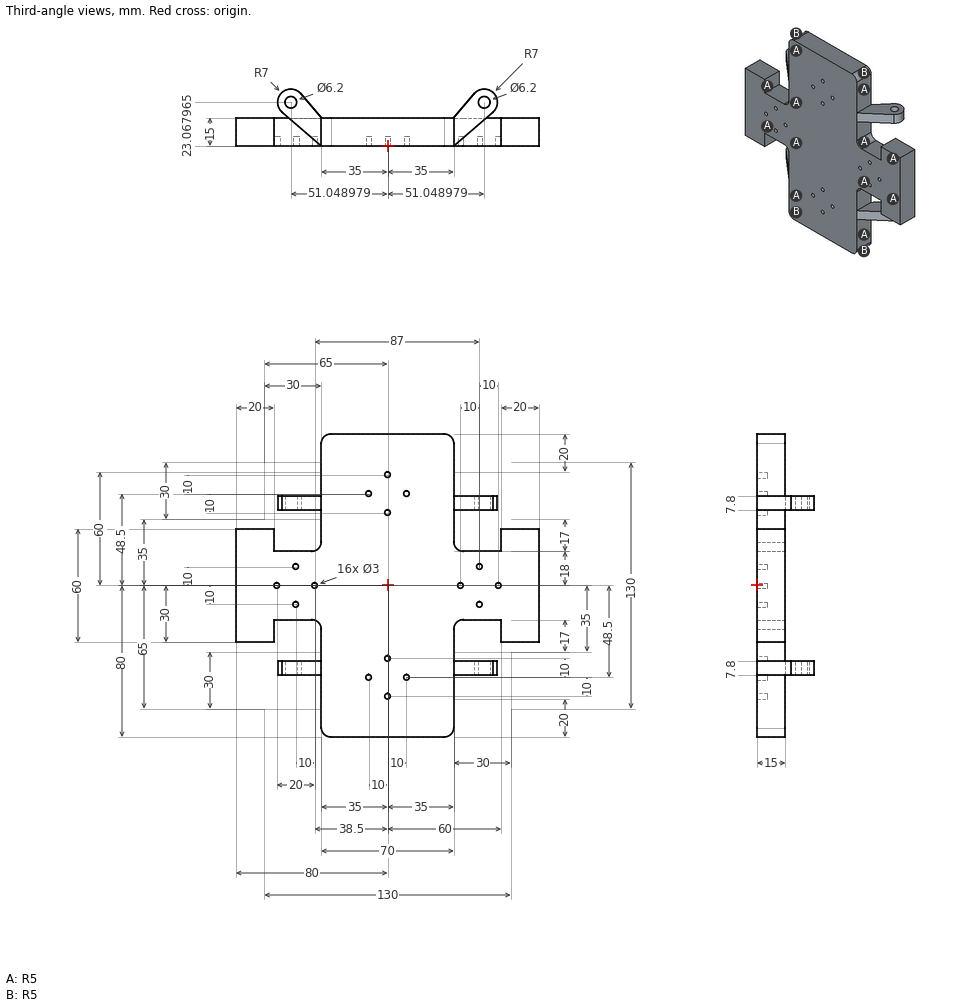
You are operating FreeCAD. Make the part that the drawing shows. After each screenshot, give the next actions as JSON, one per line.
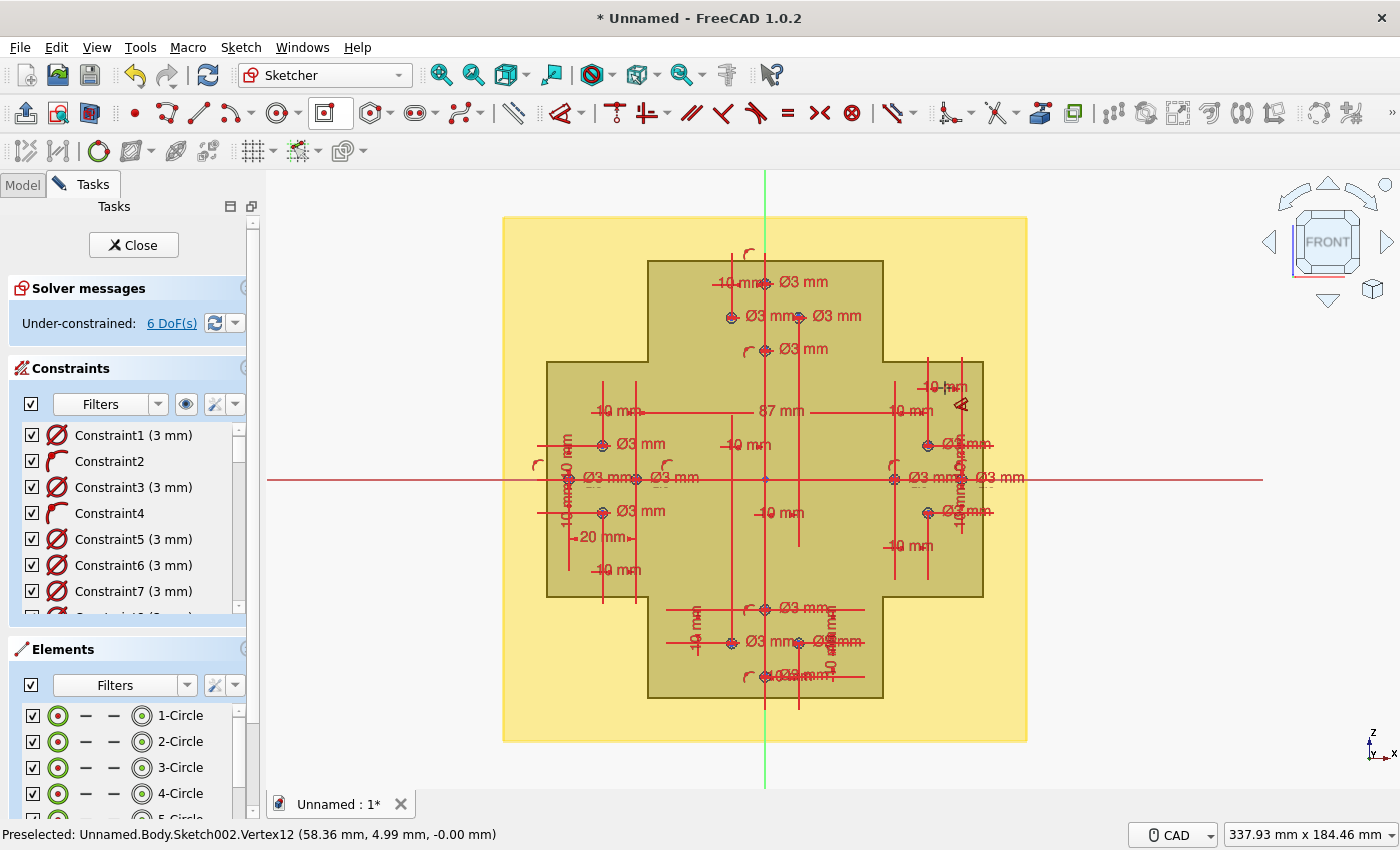
{"action": "left_click", "coordinate": [732, 318]}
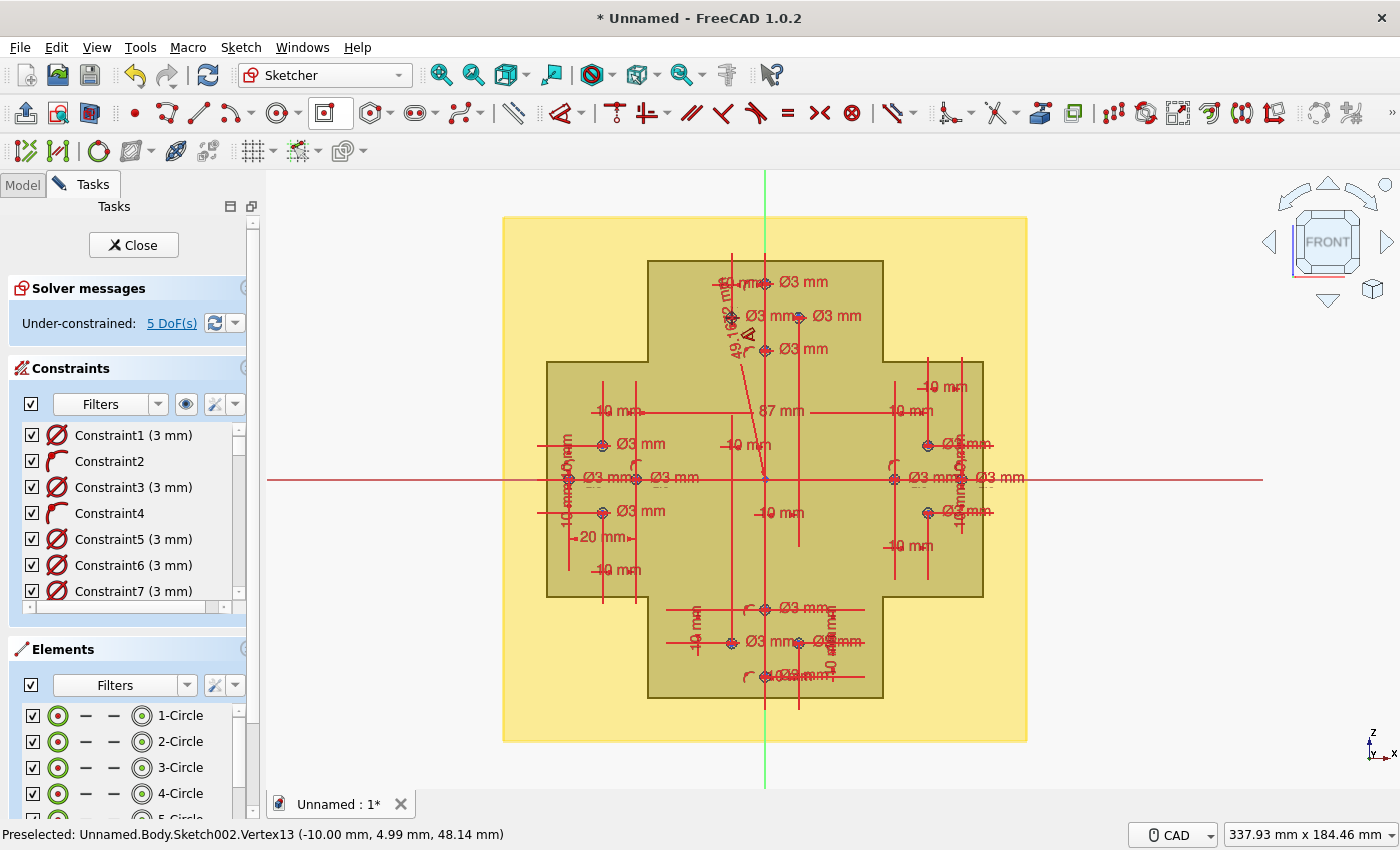
{"action": "left_click", "coordinate": [765, 351]}
{"action": "left_click", "coordinate": [698, 335]}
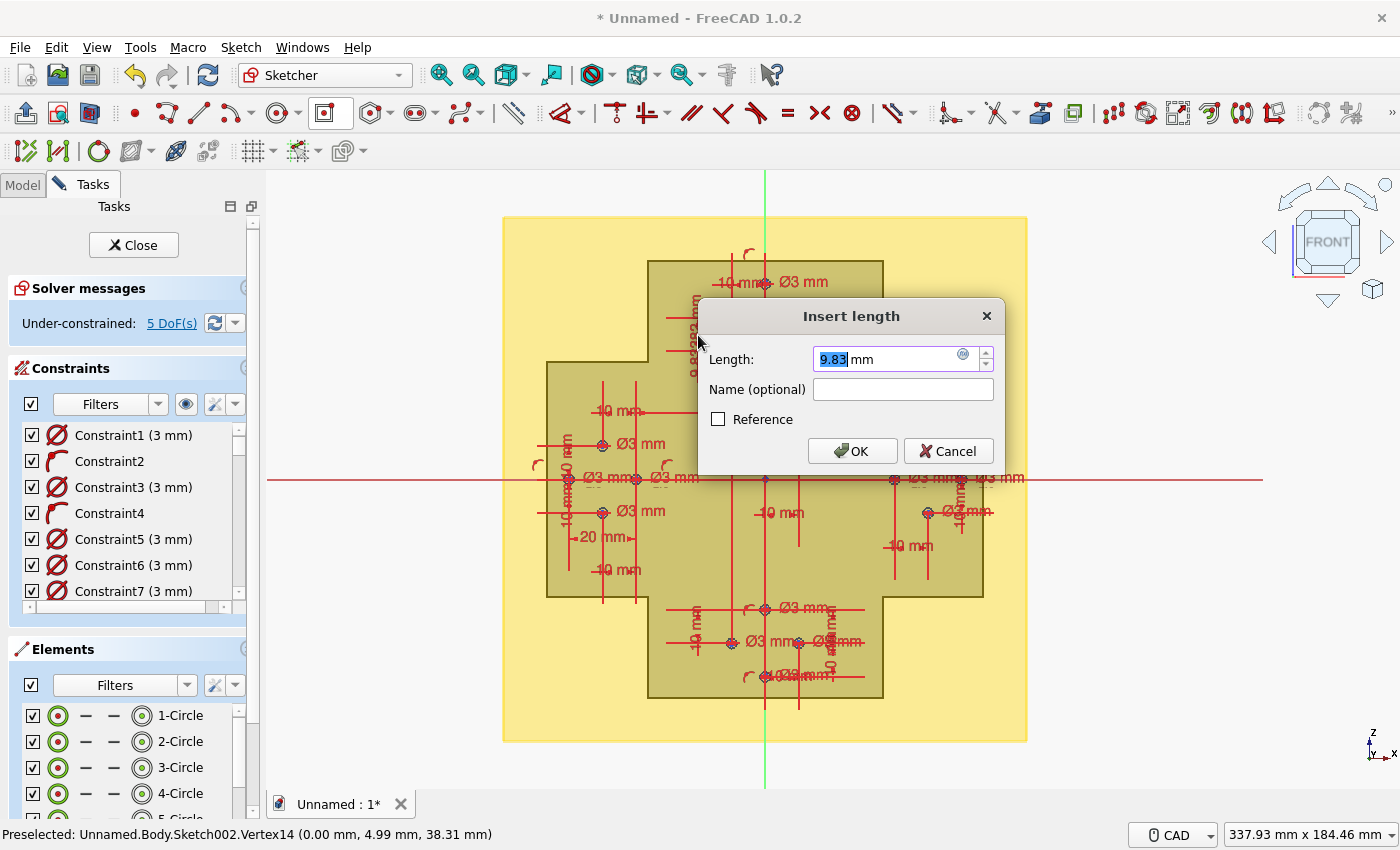
{"action": "type", "text": "10"}
{"action": "key", "text": "Return"}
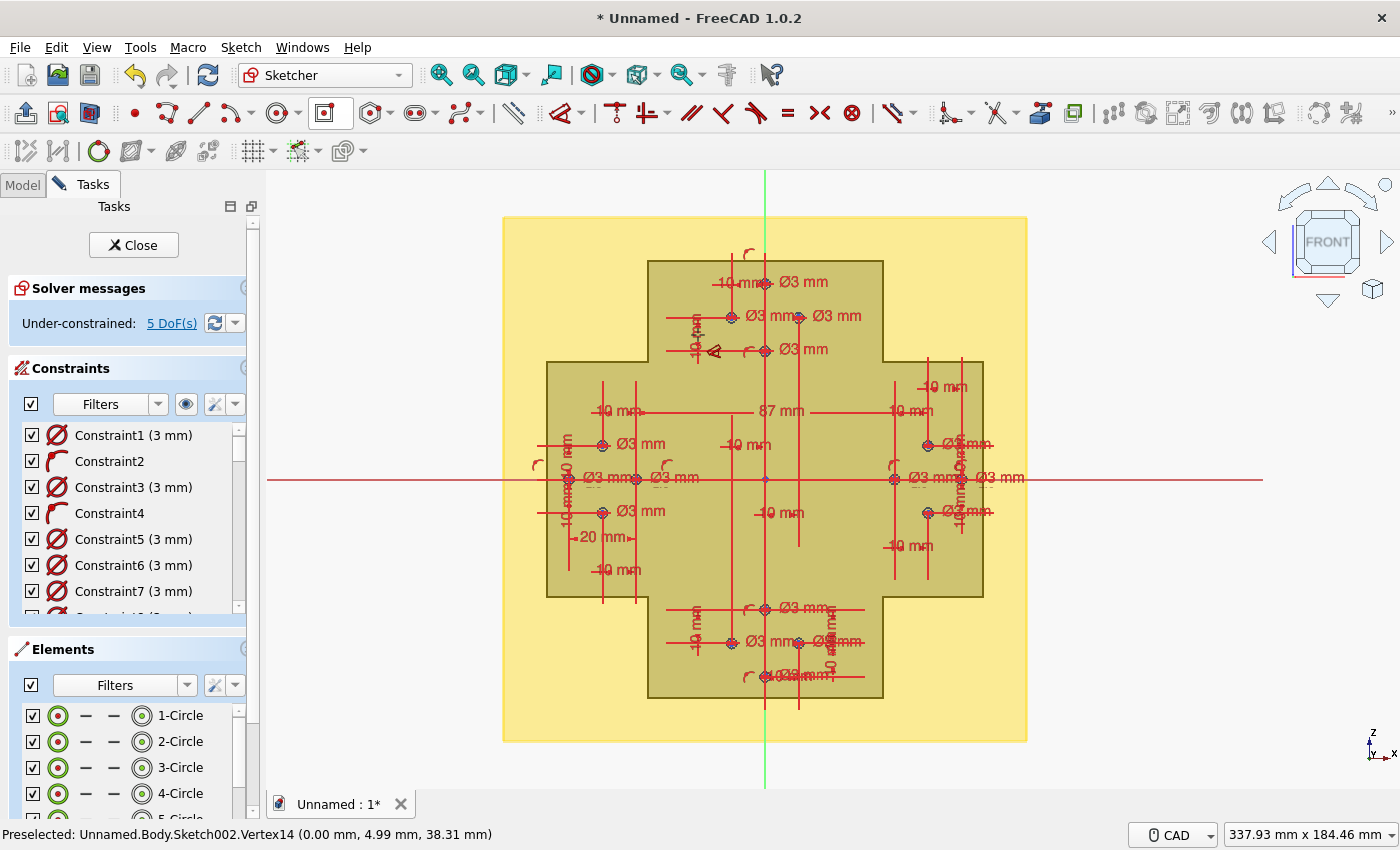
{"action": "left_click", "coordinate": [765, 351]}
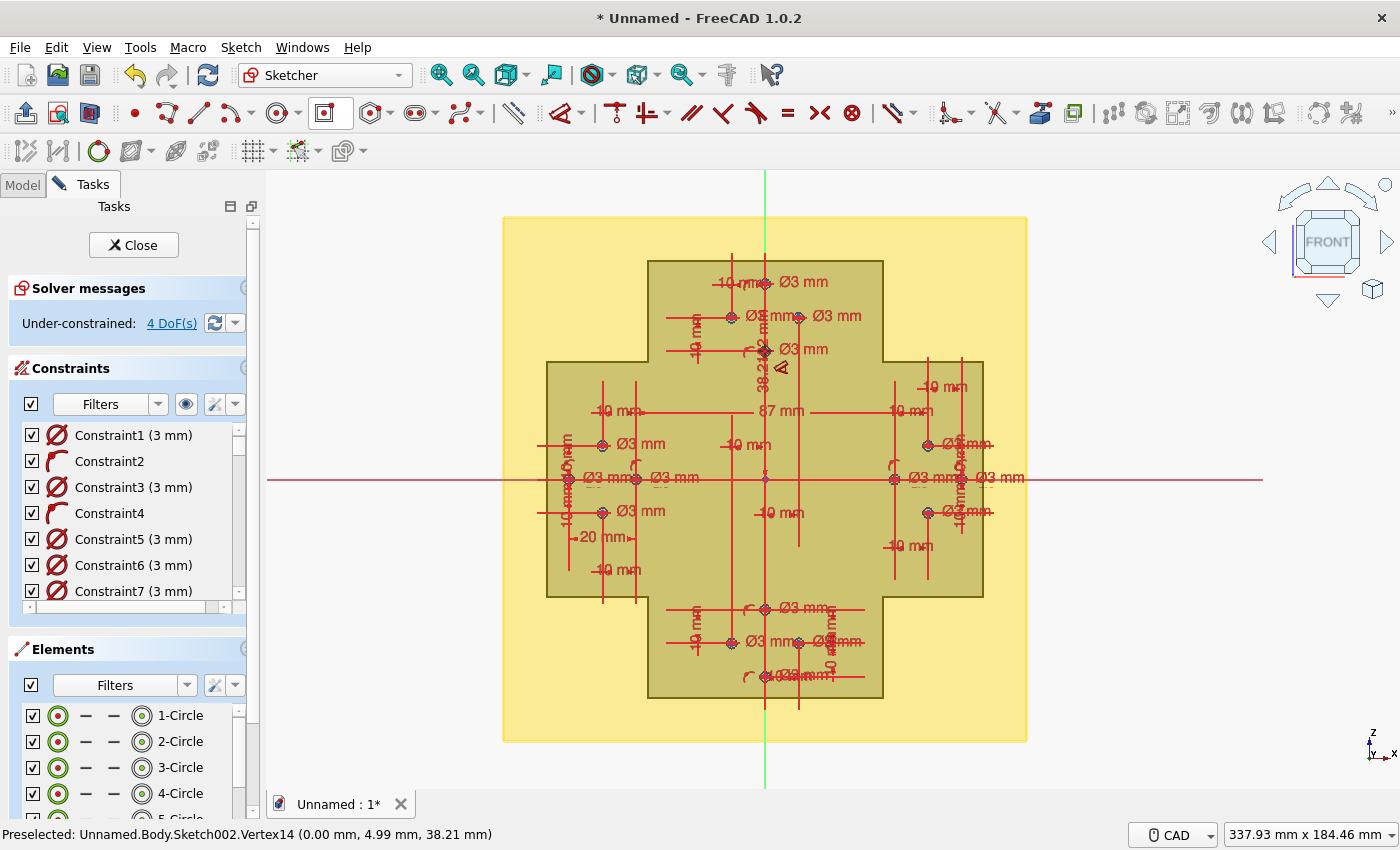
{"action": "left_click", "coordinate": [799, 318]}
{"action": "left_click", "coordinate": [833, 335]}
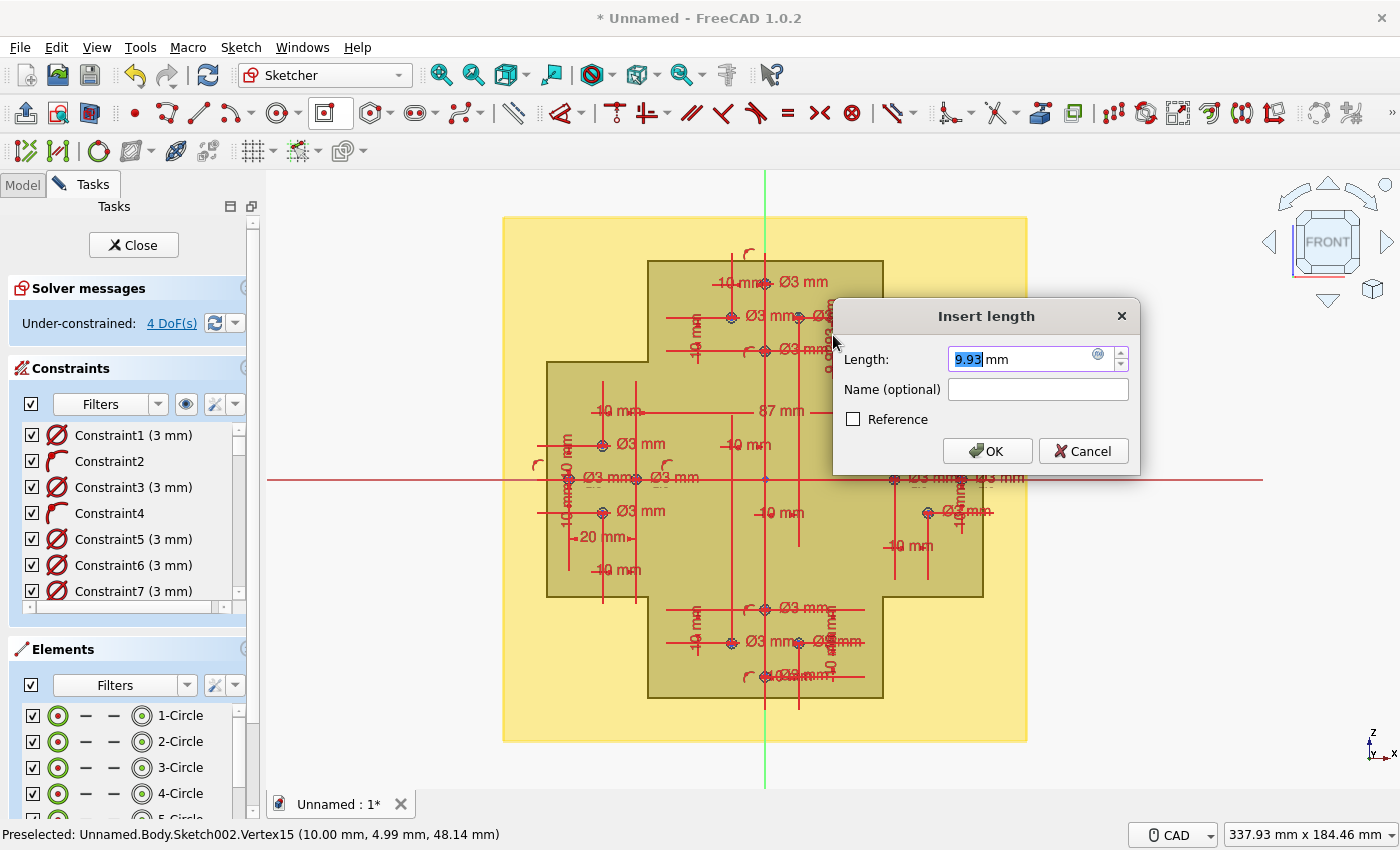
{"action": "type", "text": "10"}
{"action": "key", "text": "Return"}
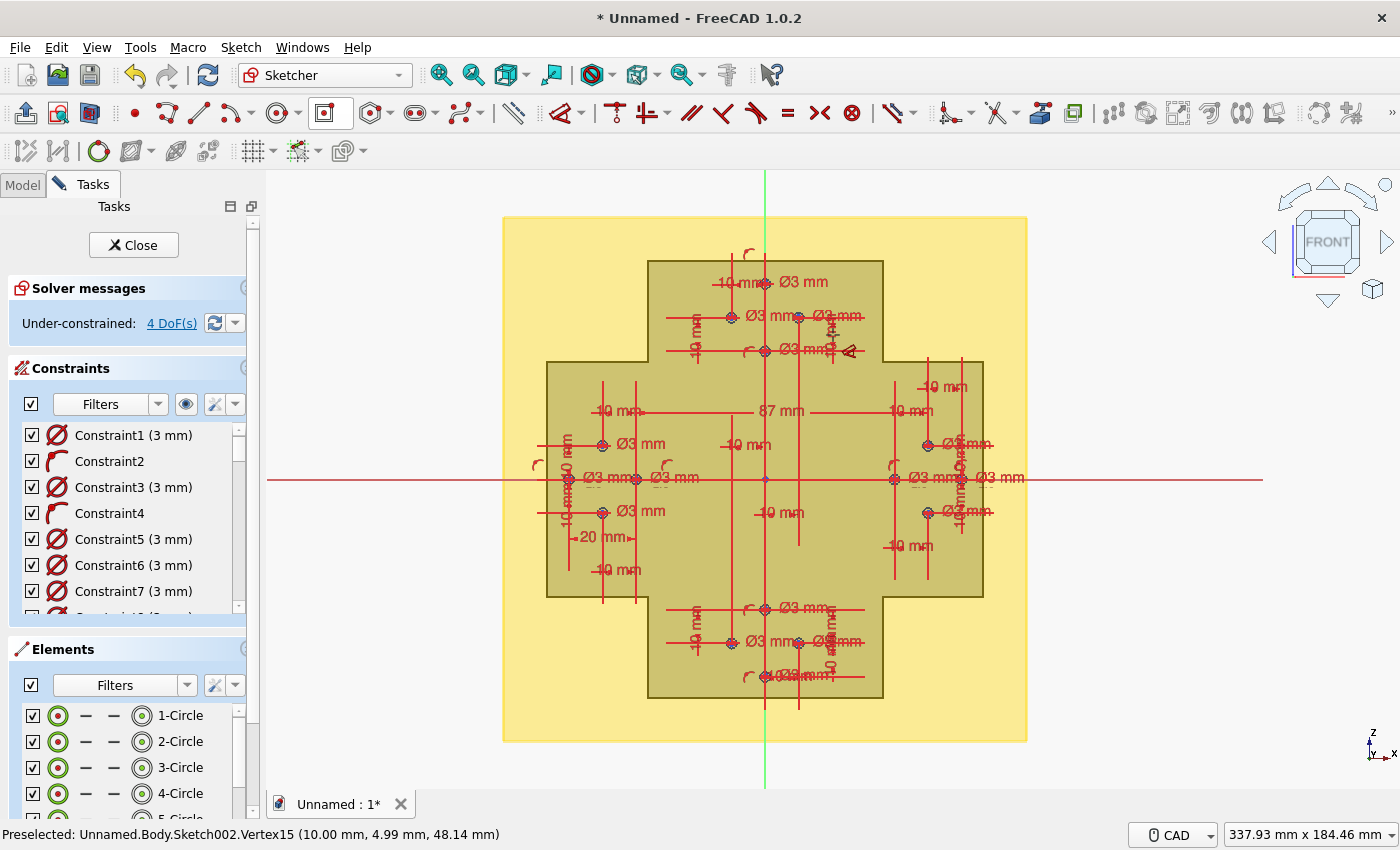
{"action": "left_click", "coordinate": [732, 318]}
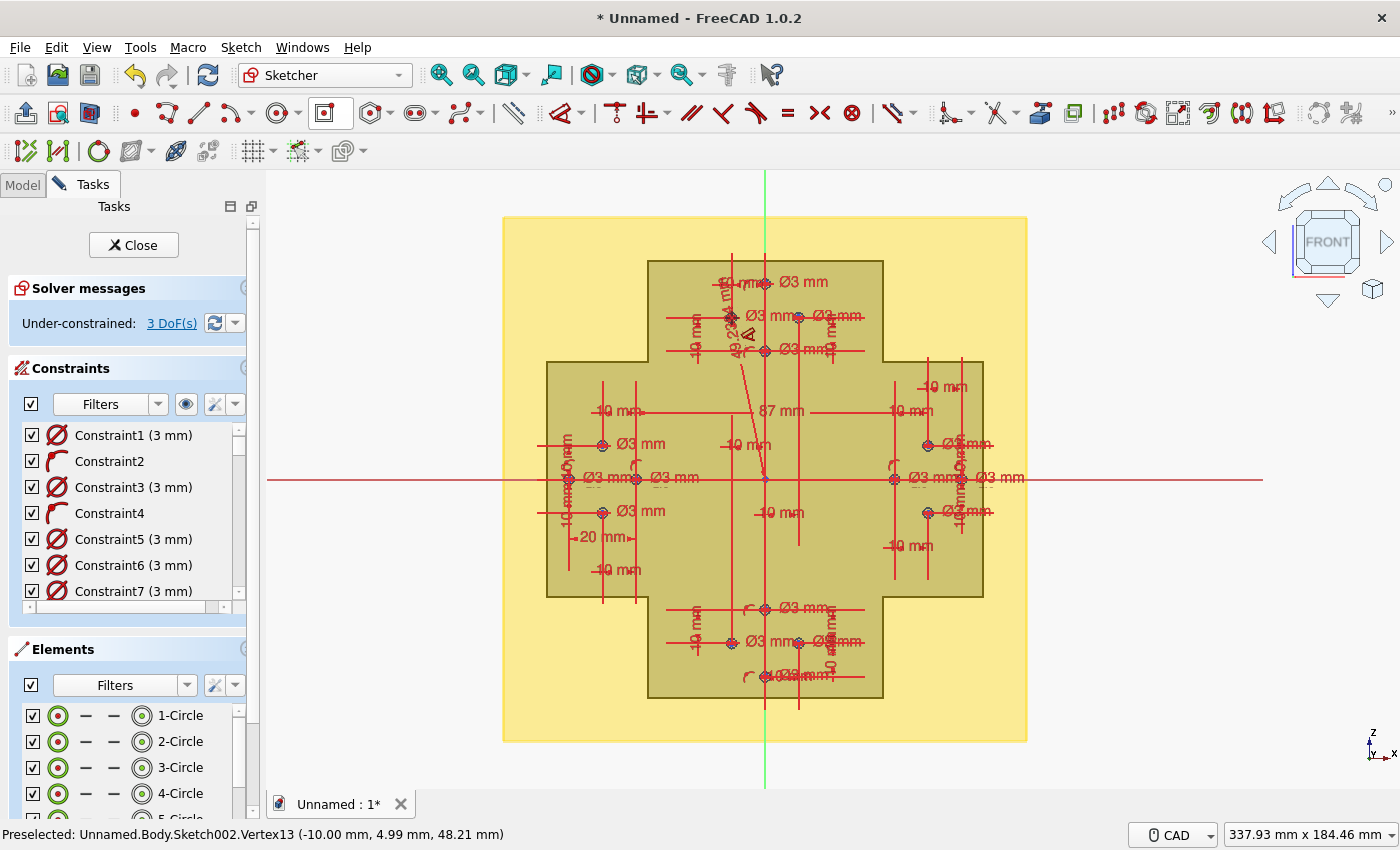
{"action": "left_click", "coordinate": [765, 284]}
{"action": "left_click", "coordinate": [698, 309]}